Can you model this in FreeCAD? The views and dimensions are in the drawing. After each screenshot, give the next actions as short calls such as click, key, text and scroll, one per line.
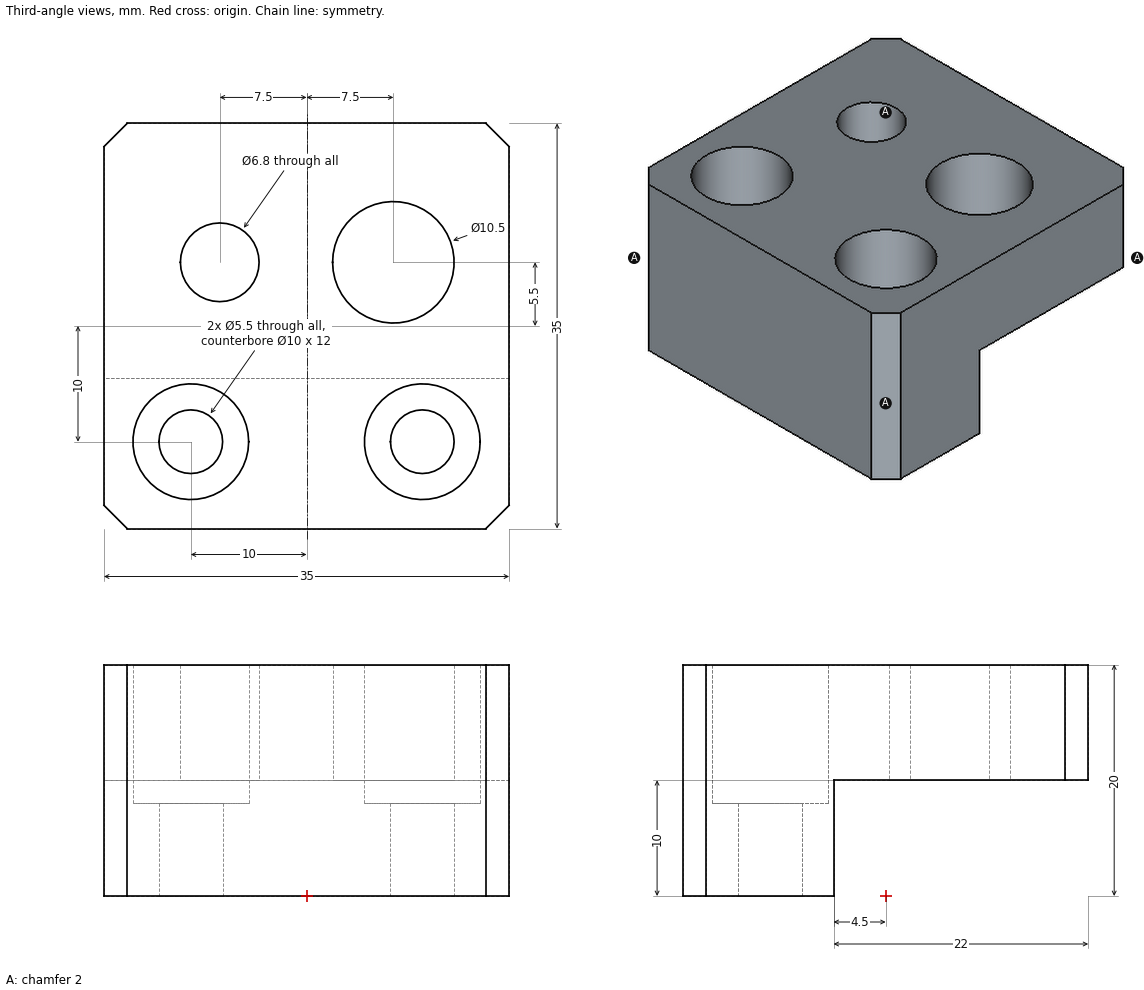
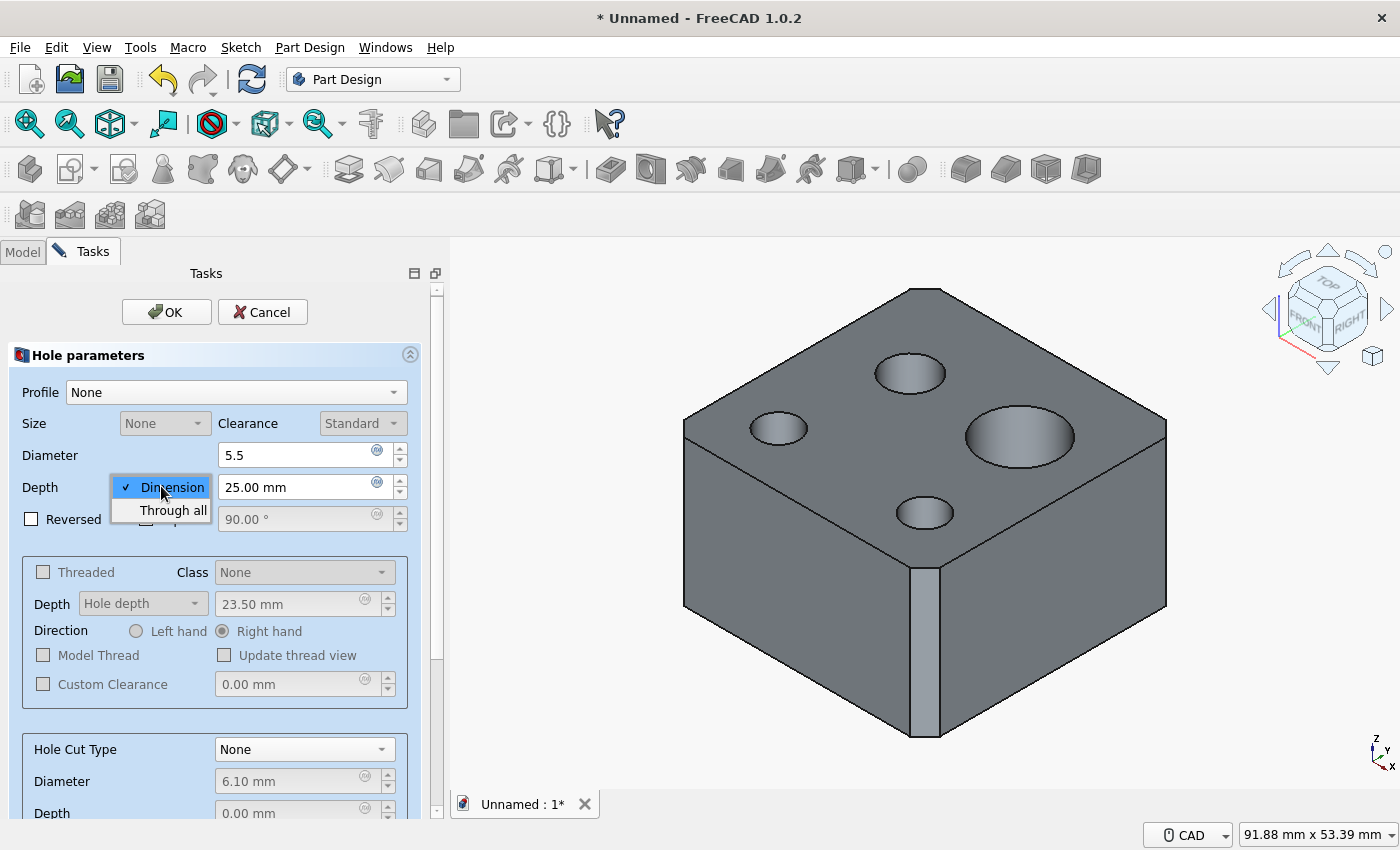
click(160, 510)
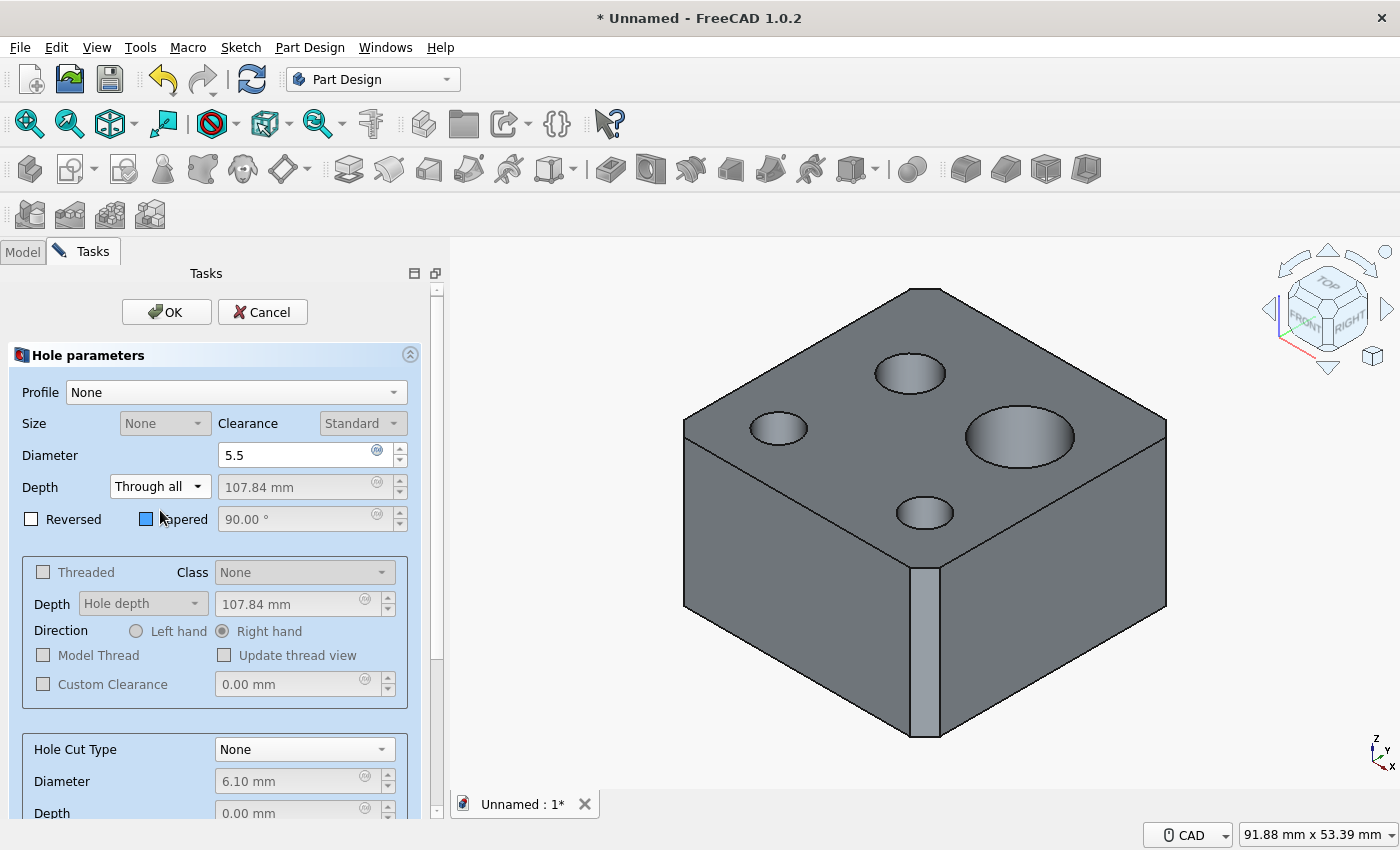
click(306, 750)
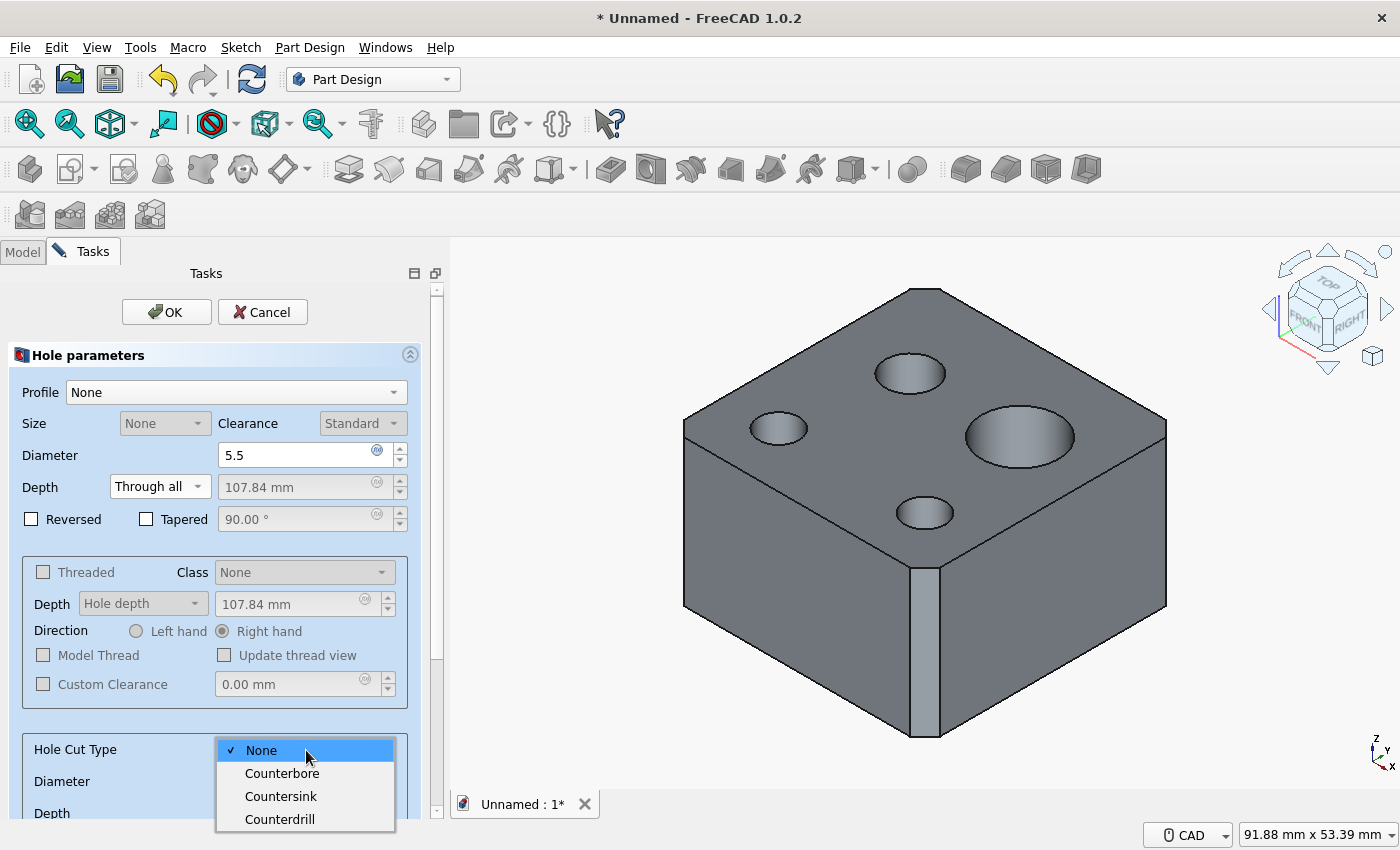
click(304, 774)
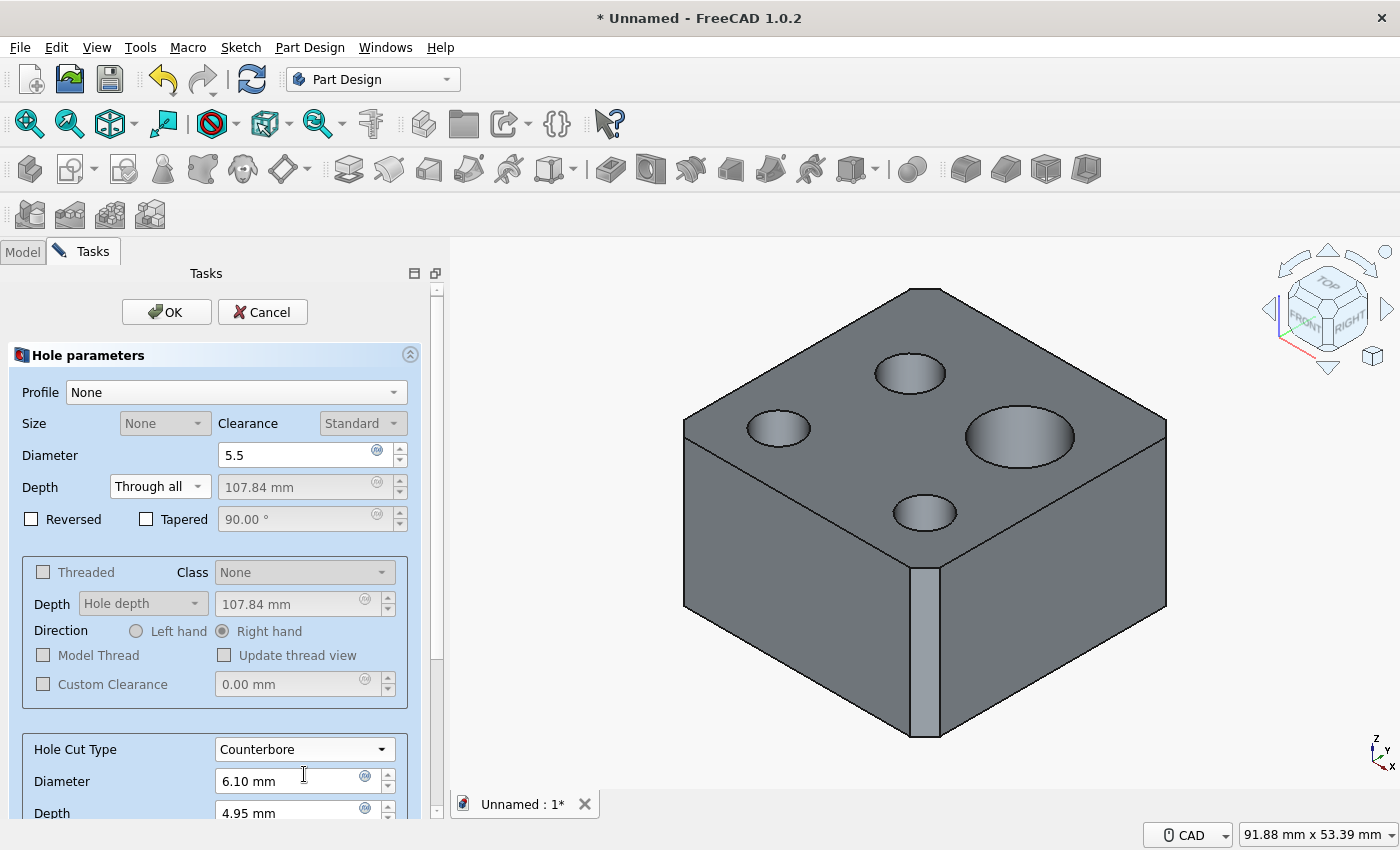
triple_click(298, 781)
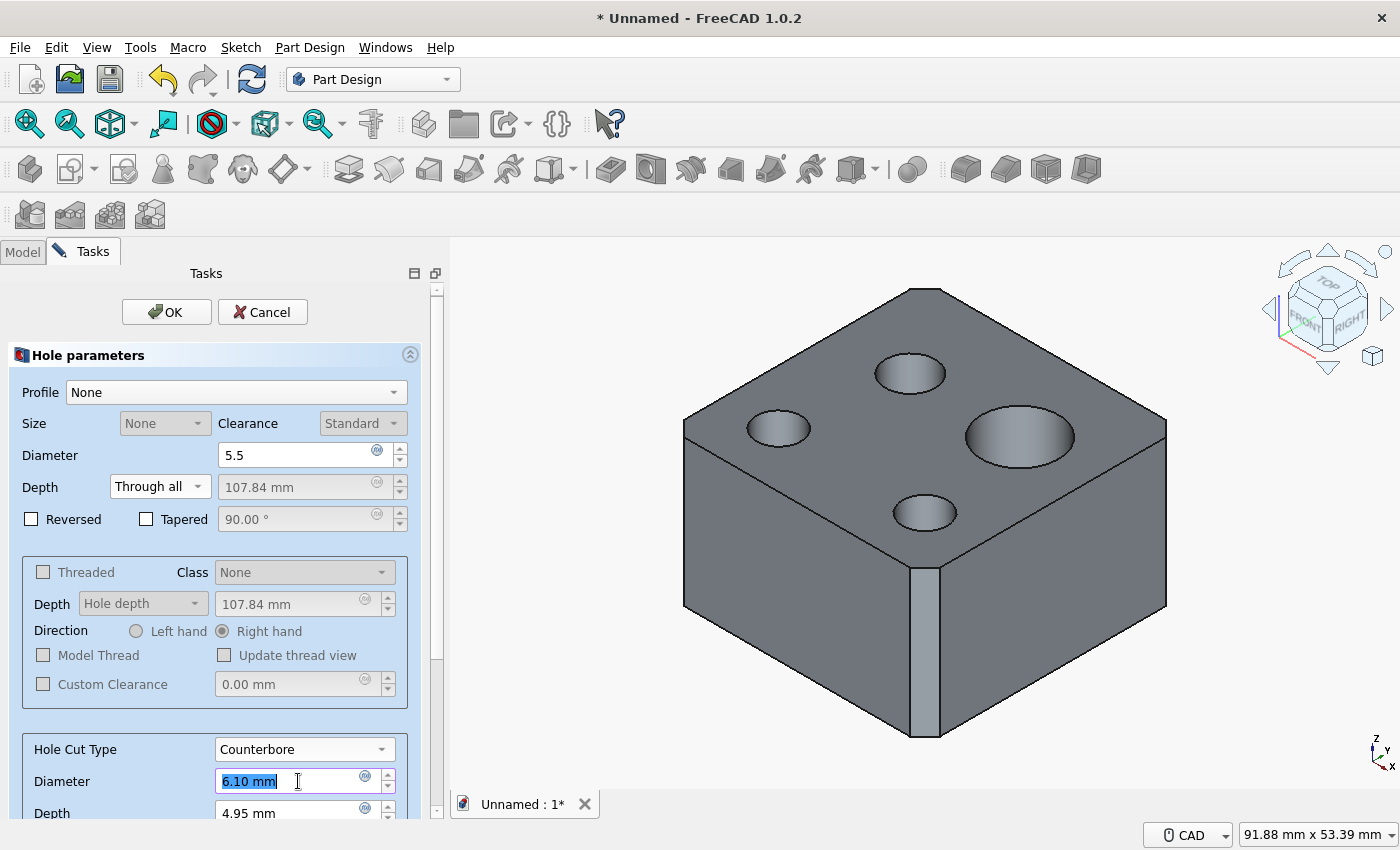
text(10)
key(Tab)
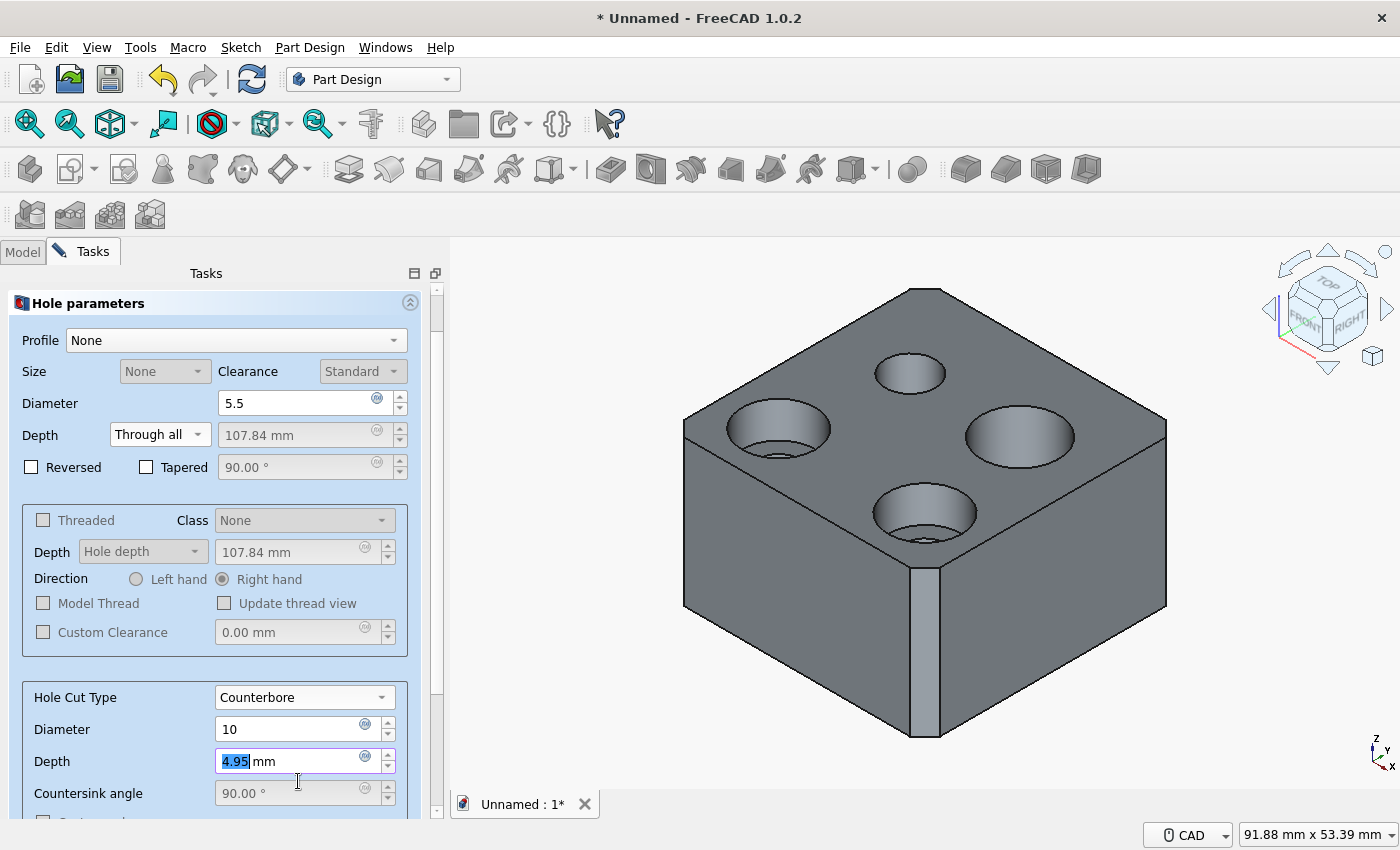
text(12)
key(Tab)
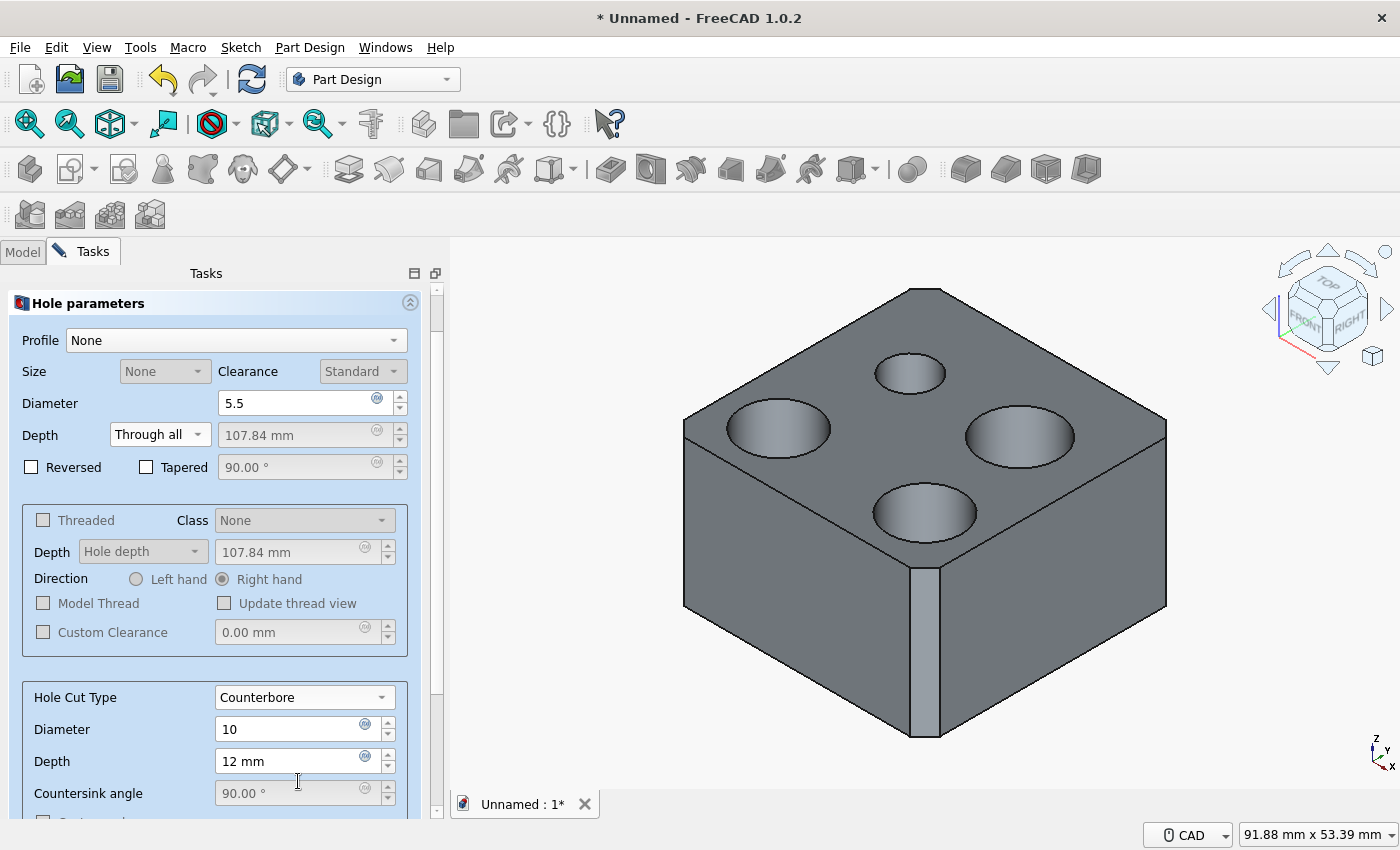
scroll(437, 550, up, 2)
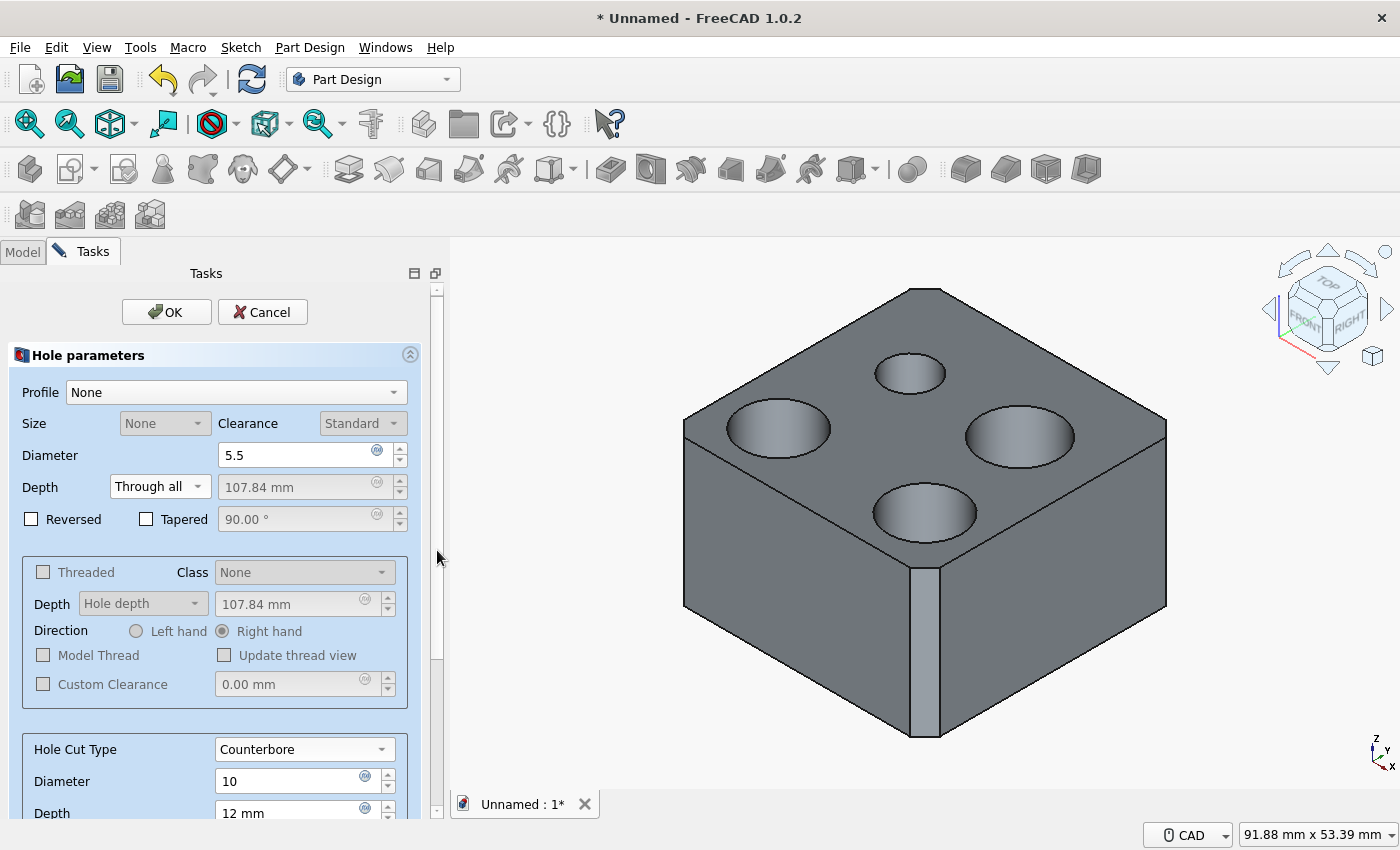
click(167, 312)